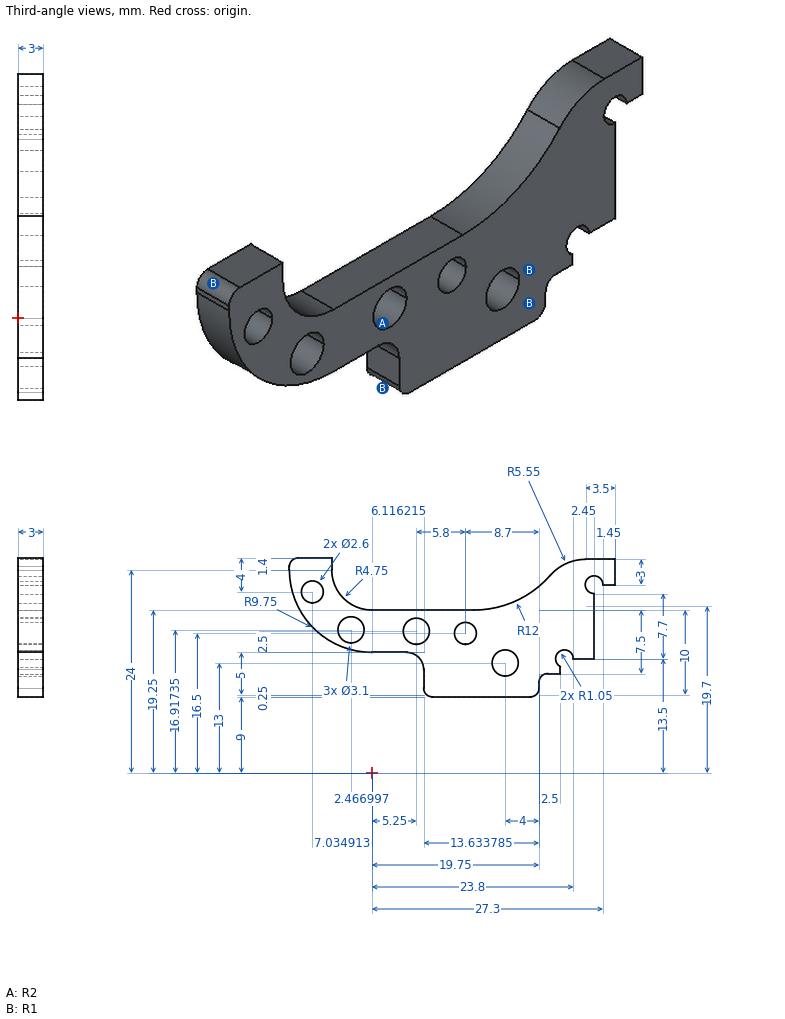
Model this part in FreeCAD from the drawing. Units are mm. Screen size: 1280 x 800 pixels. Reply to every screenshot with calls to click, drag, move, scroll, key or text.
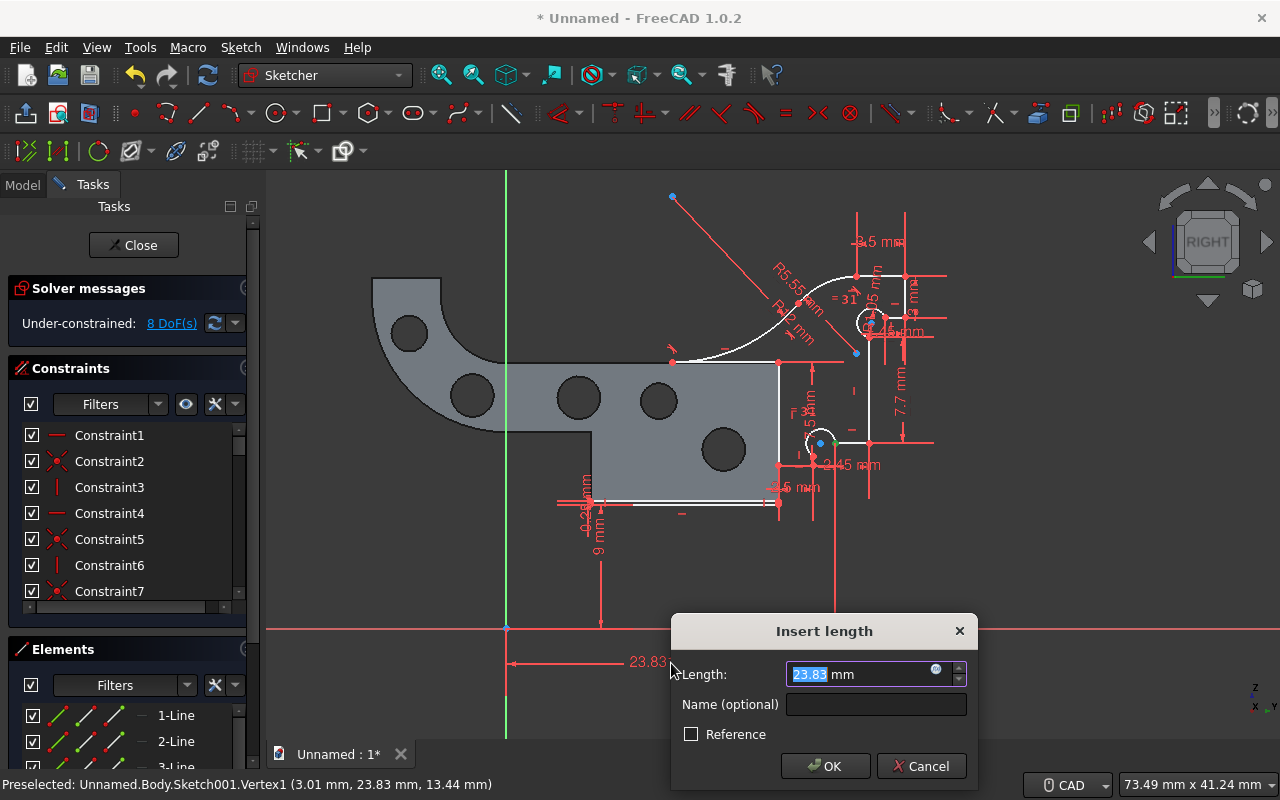
text(23.8)
key(Return)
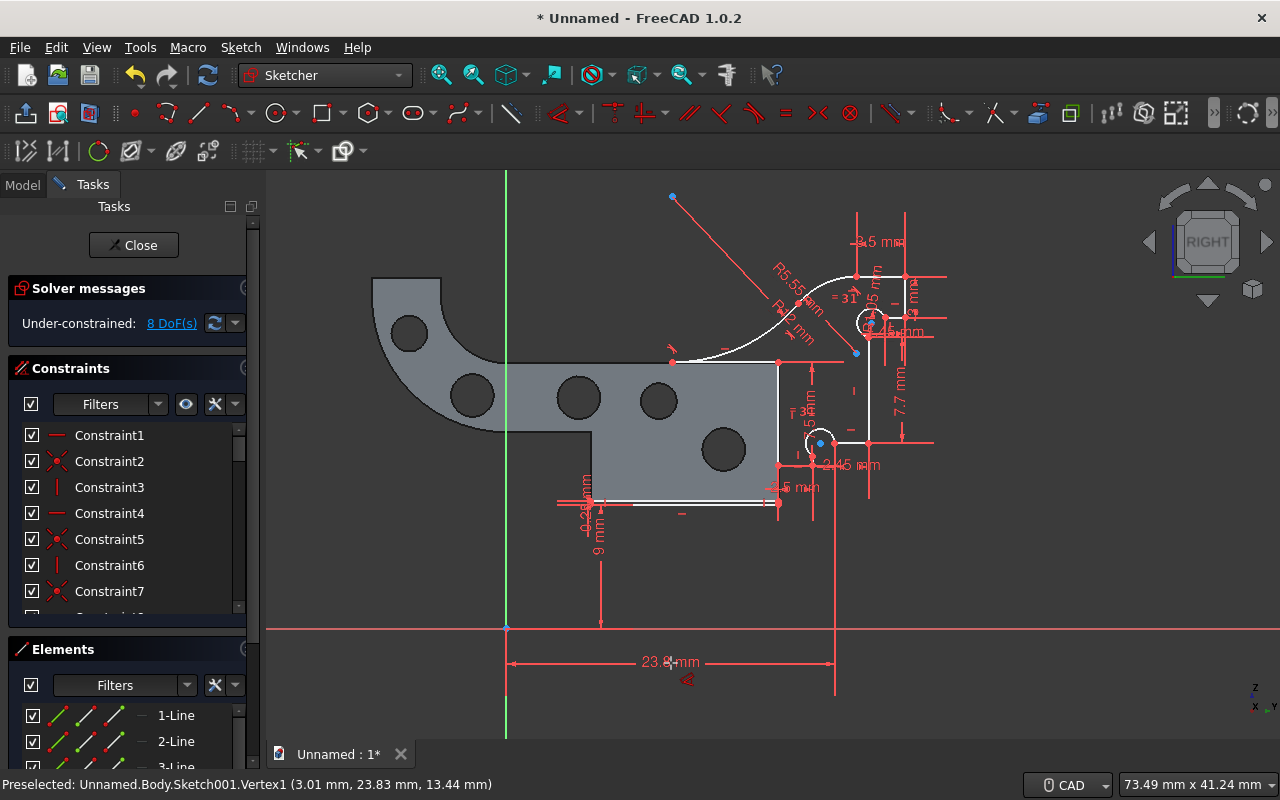
click(835, 443)
click(472, 536)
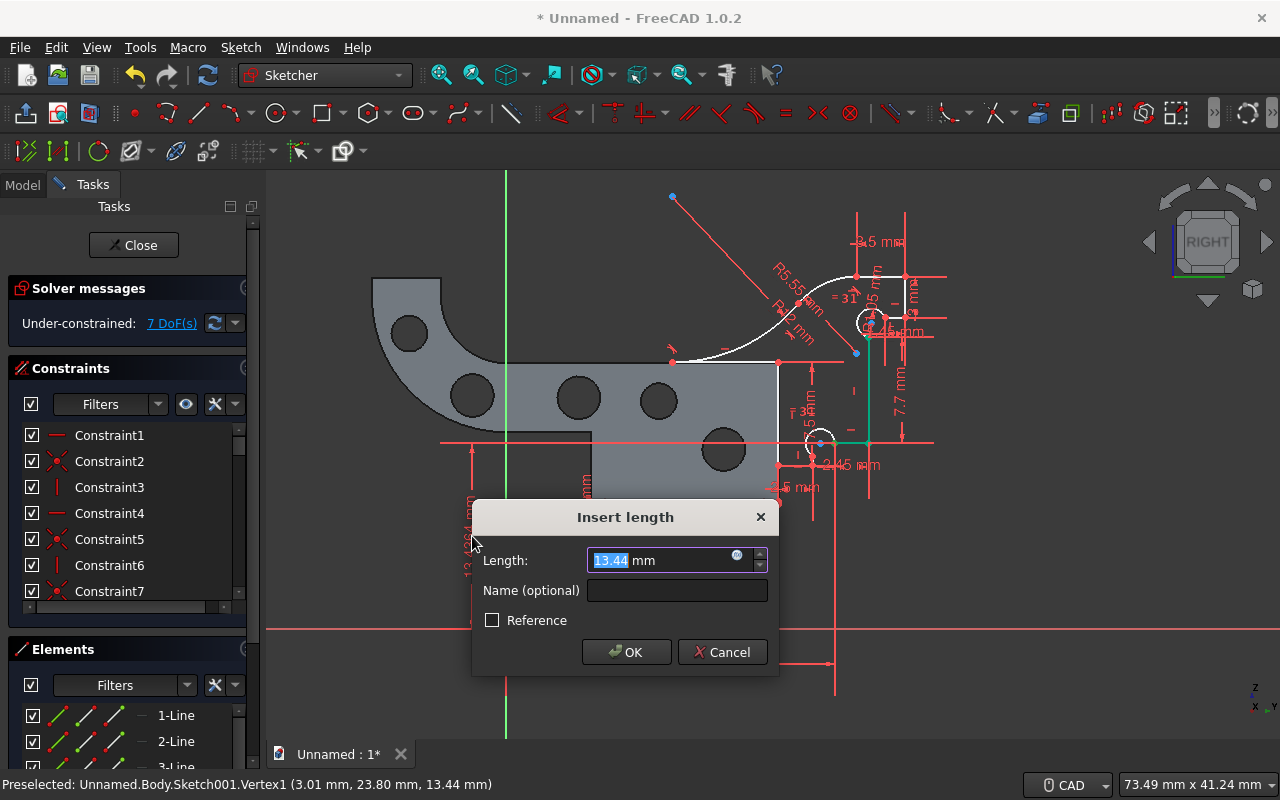
text(13.5)
key(Return)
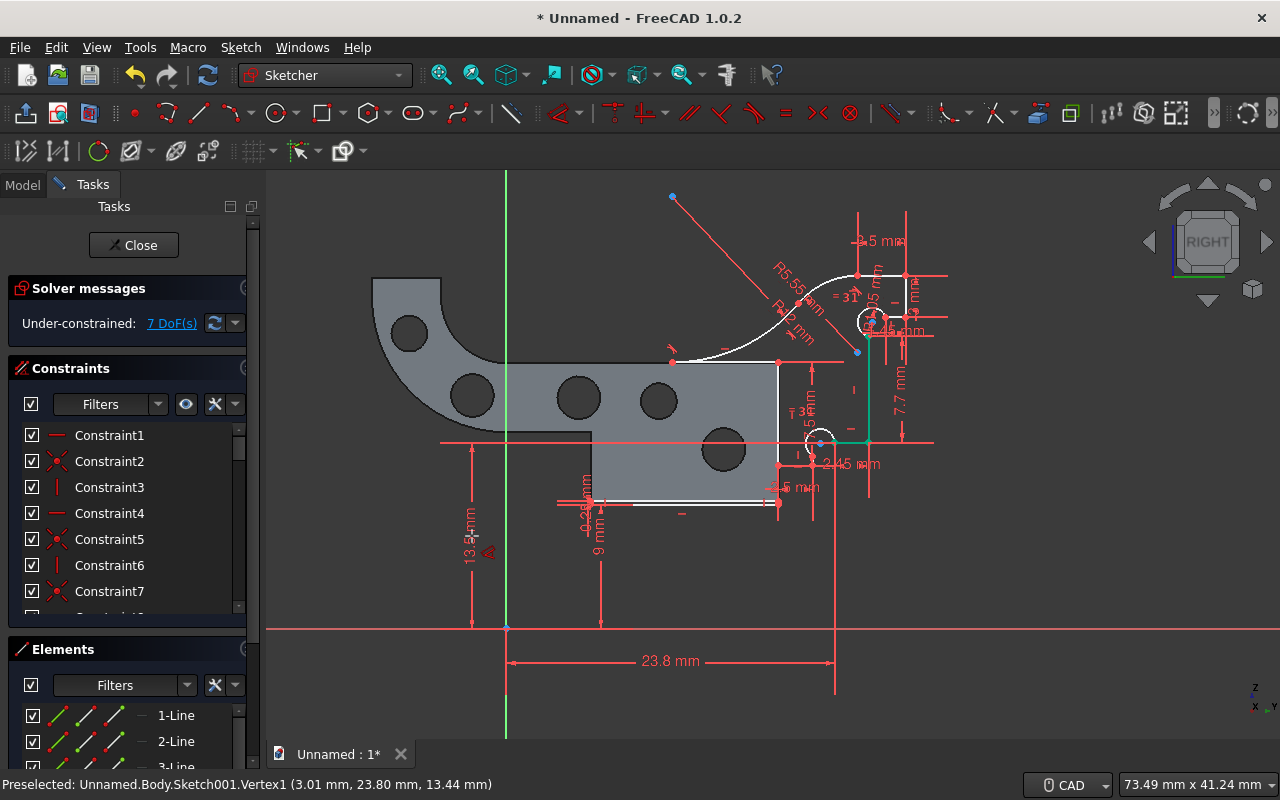
click(886, 317)
click(783, 663)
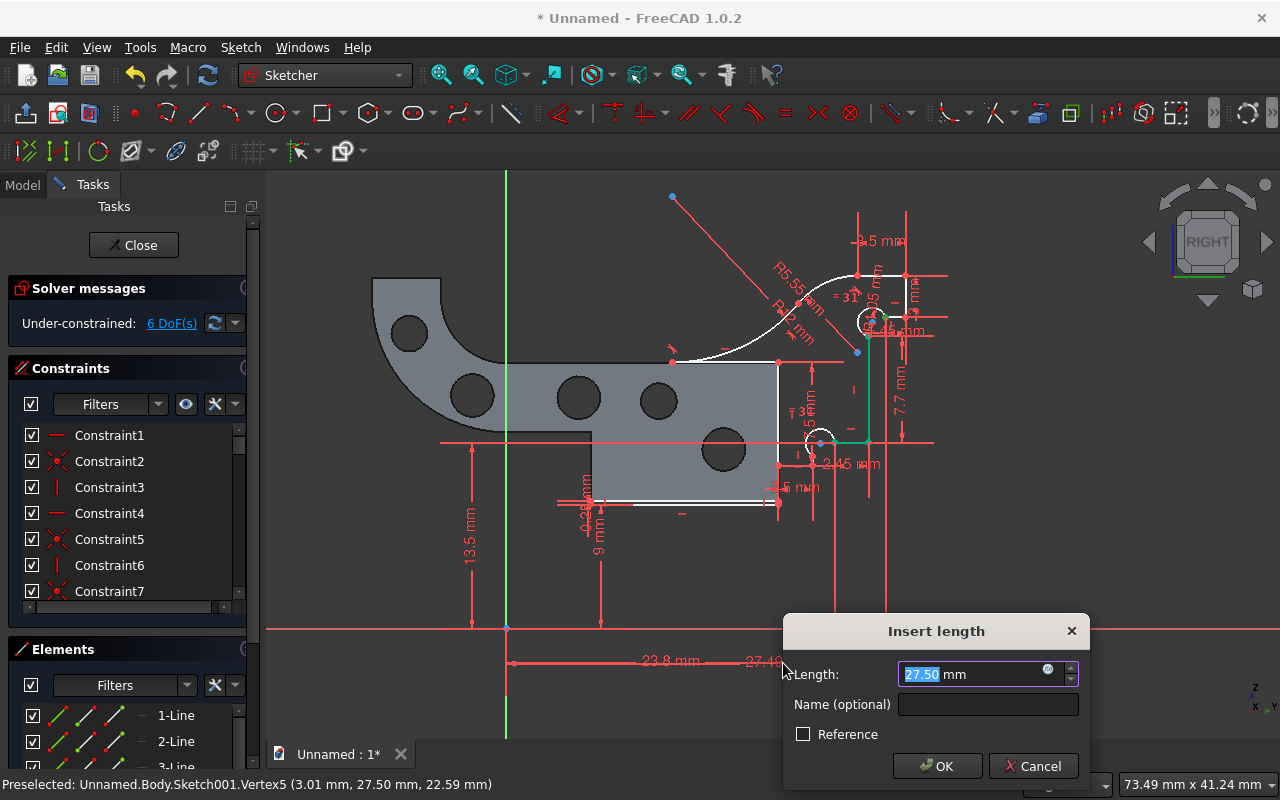
text(27.3)
key(Return)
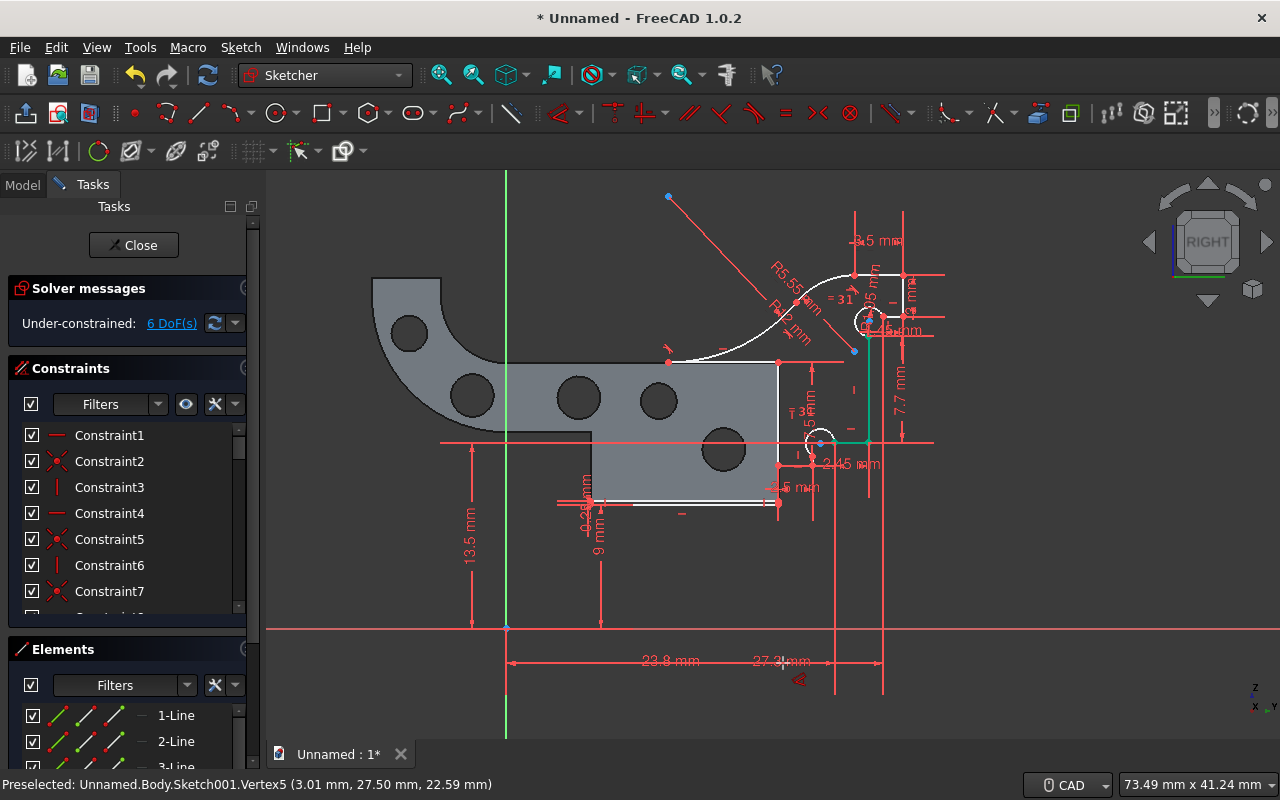
click(855, 352)
click(472, 490)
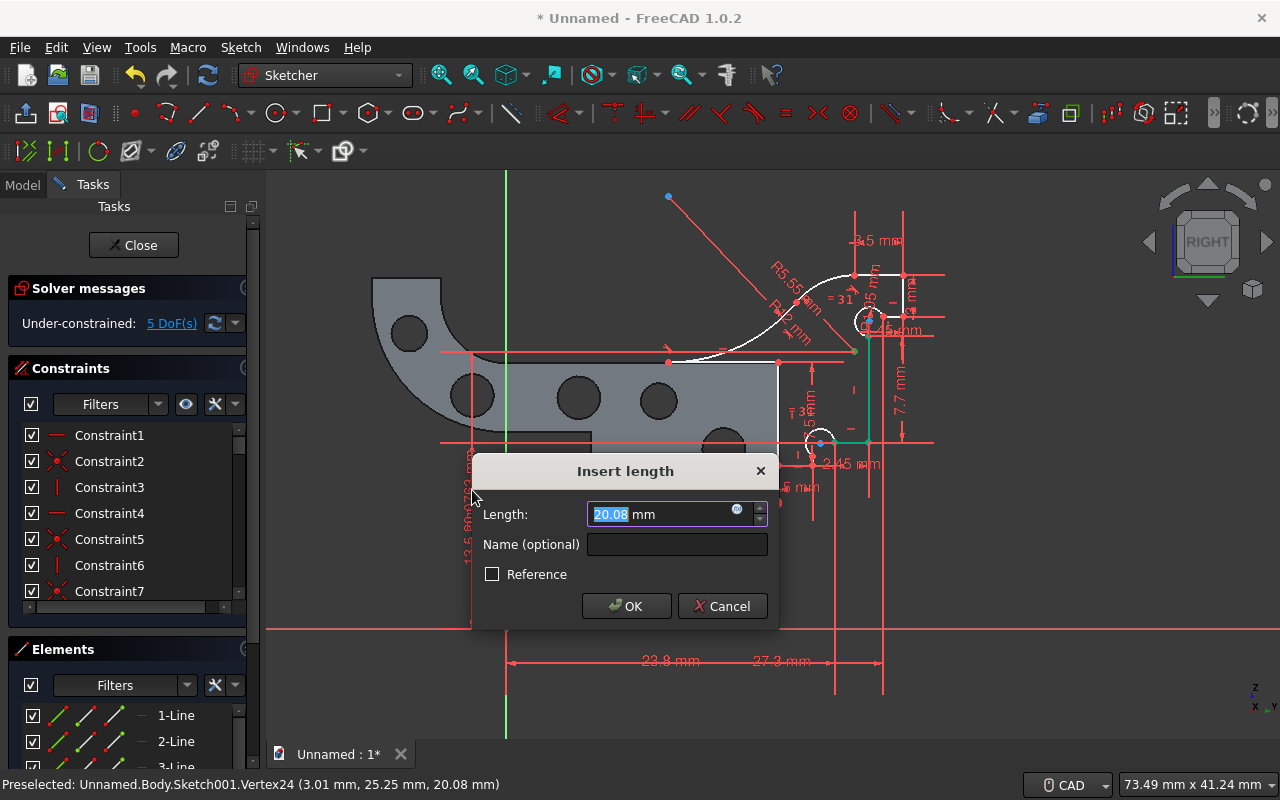
text(19.7)
key(Return)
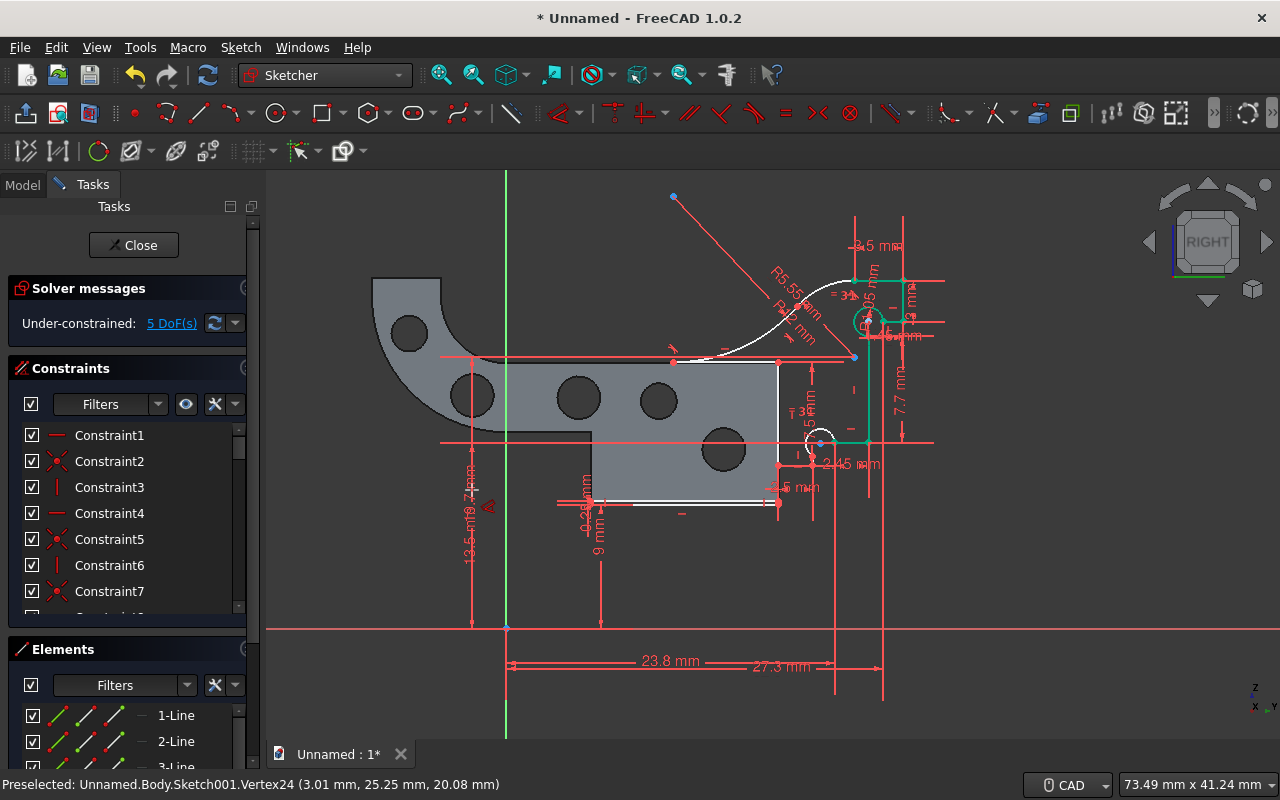
click(820, 444)
click(472, 579)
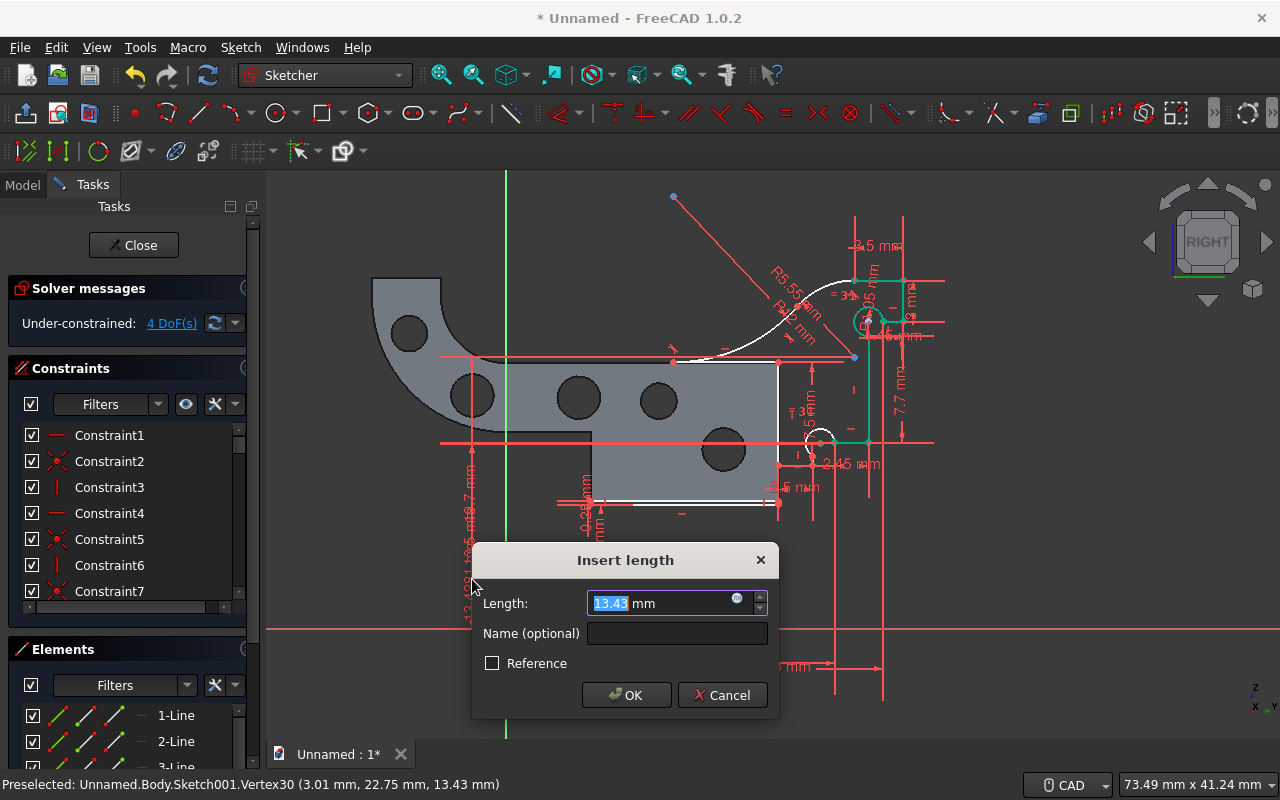
text(13.5)
key(Return)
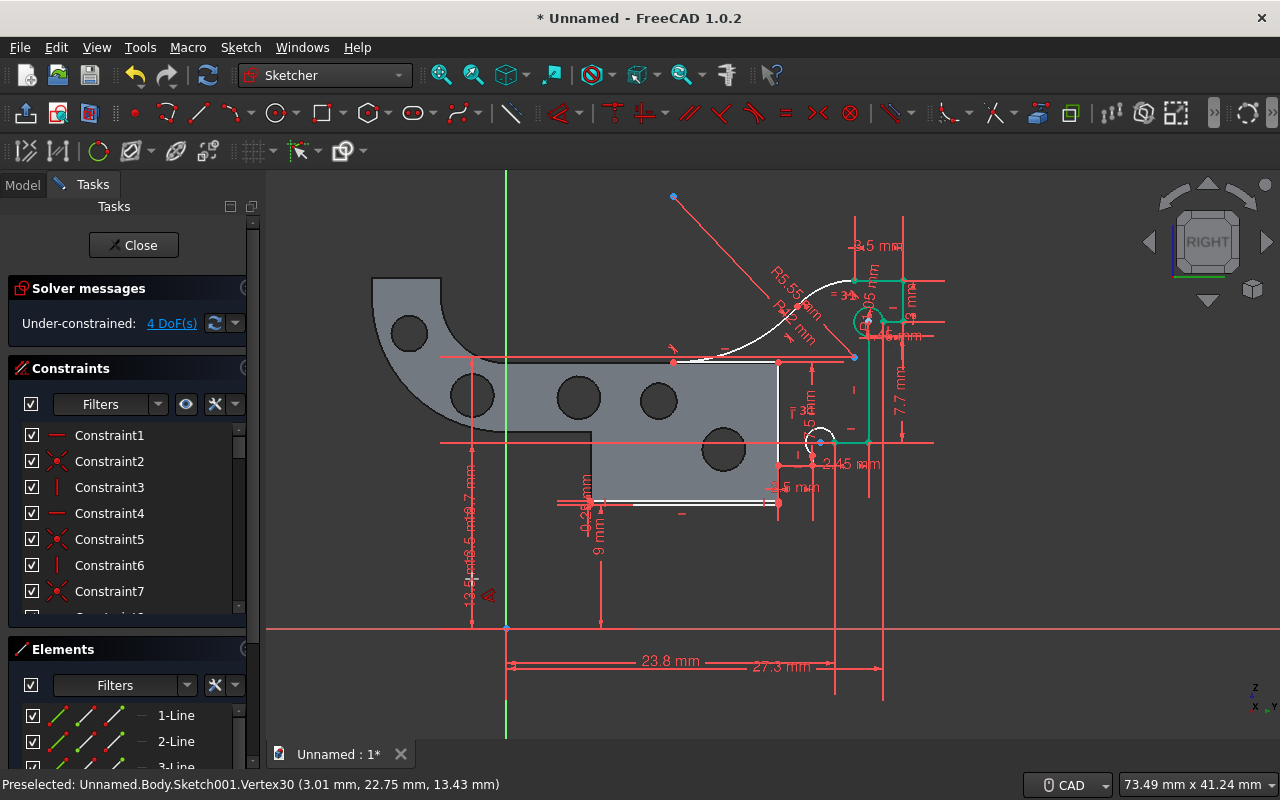
click(673, 362)
click(472, 434)